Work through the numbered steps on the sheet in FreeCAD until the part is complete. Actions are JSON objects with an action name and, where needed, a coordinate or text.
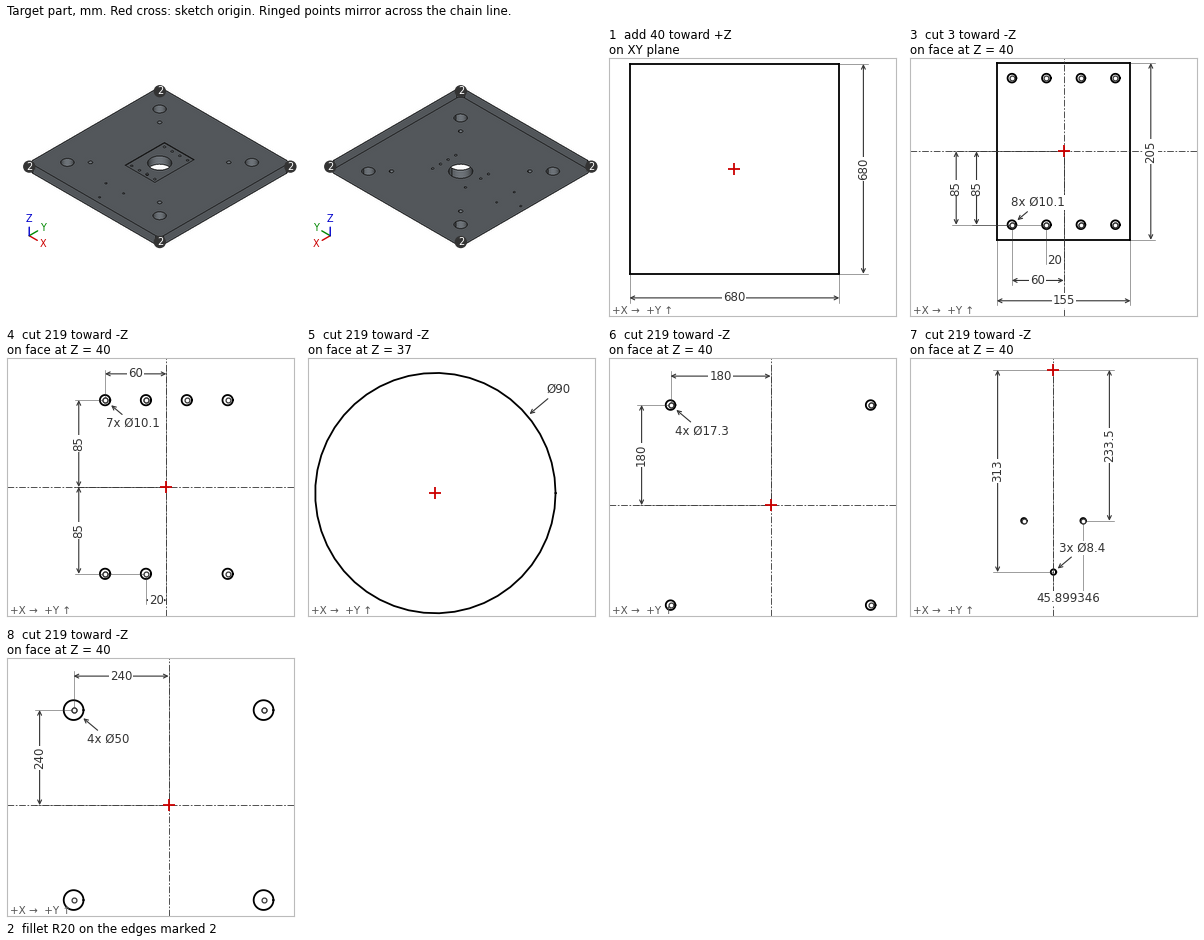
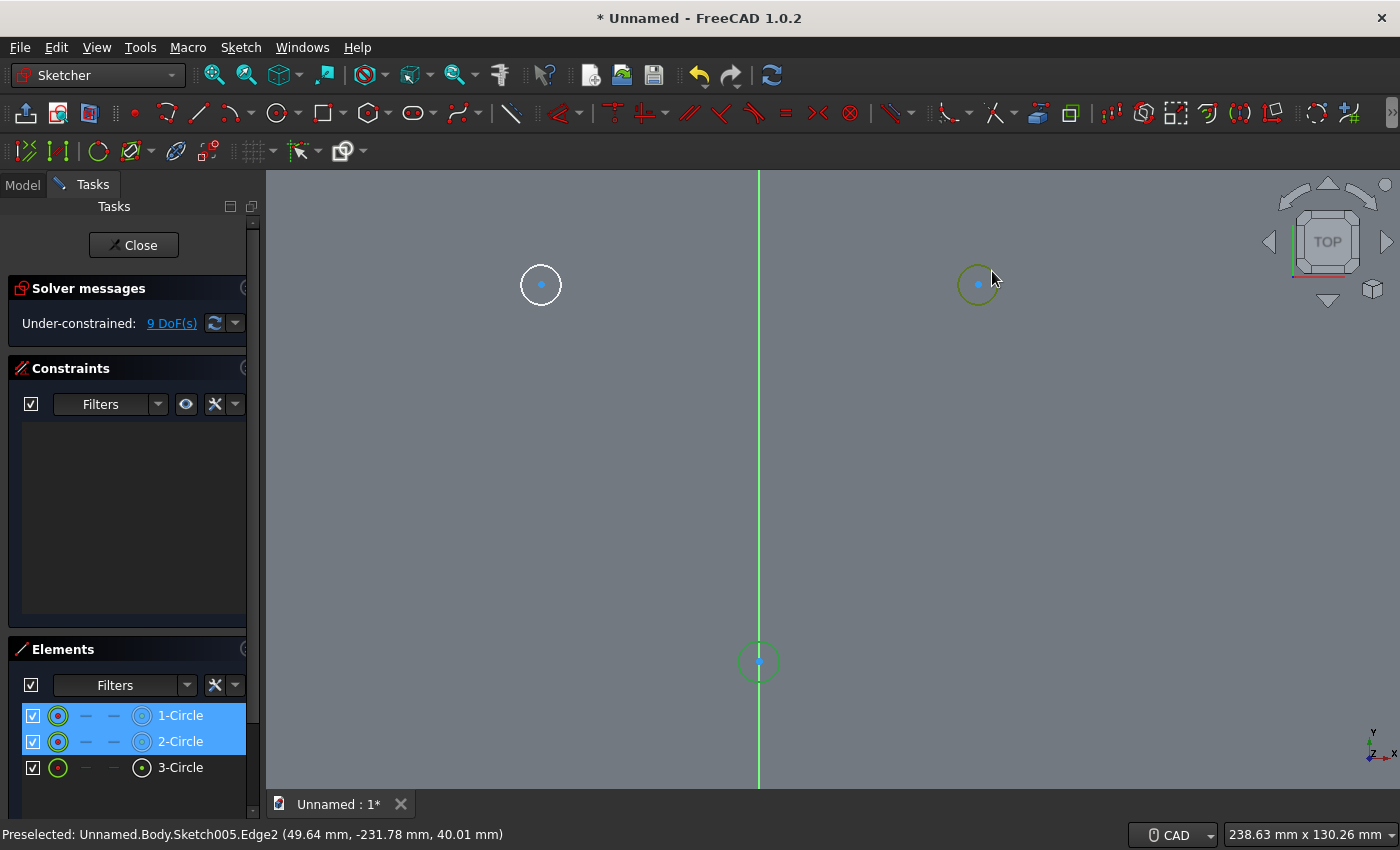
{"action": "left_click", "coordinate": [555, 271]}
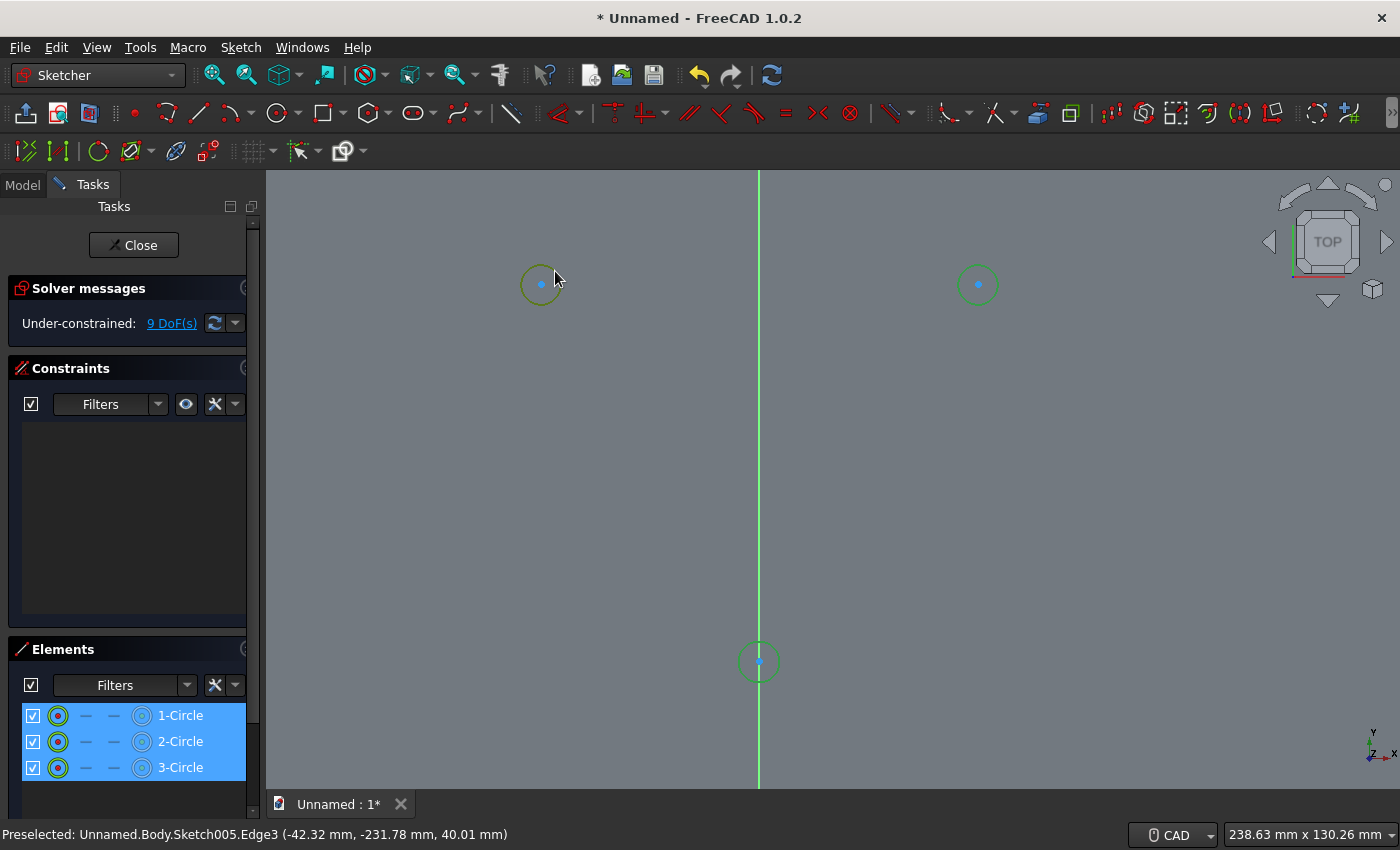
{"action": "left_click", "coordinate": [786, 114]}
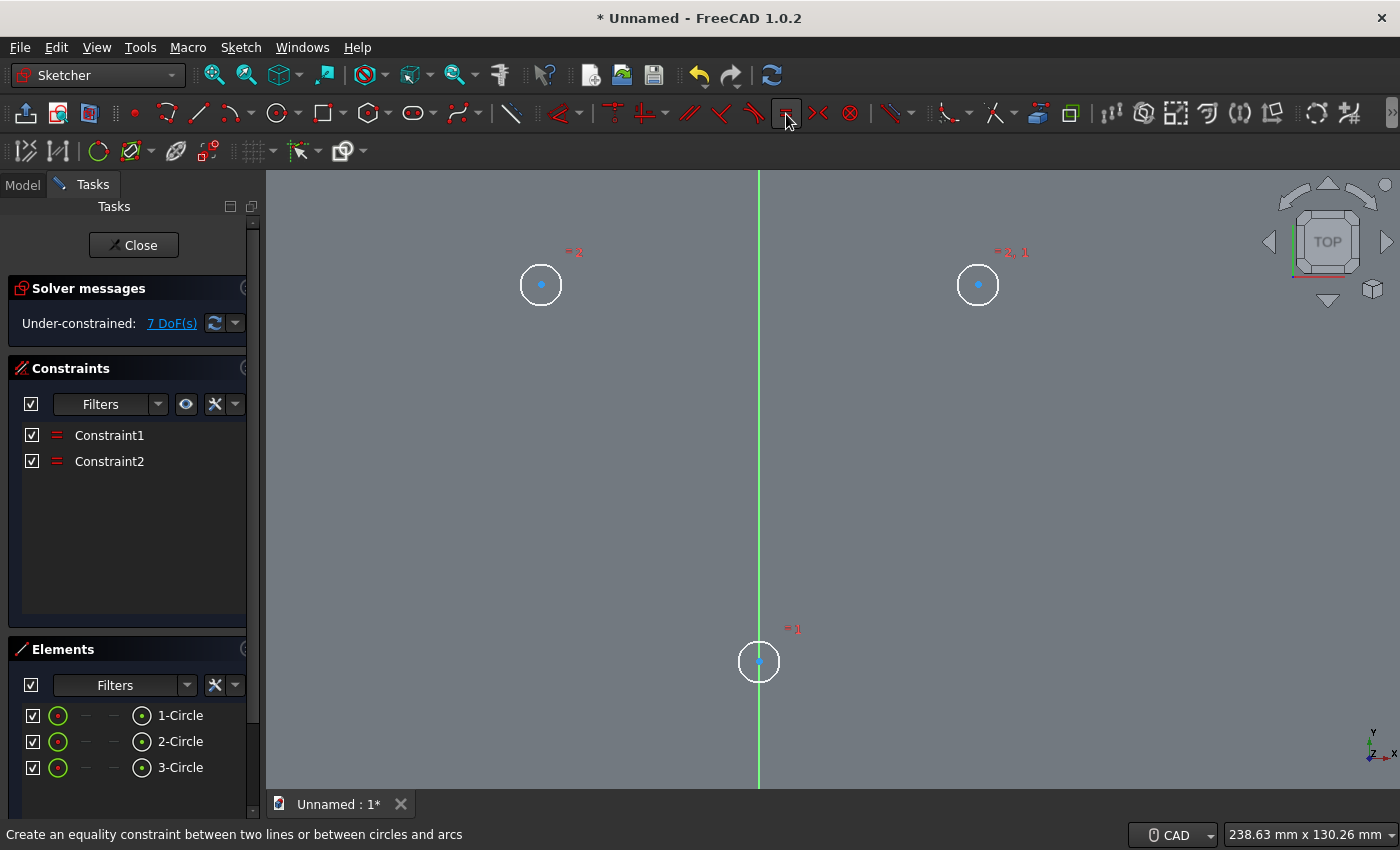
{"action": "left_click", "coordinate": [759, 662]}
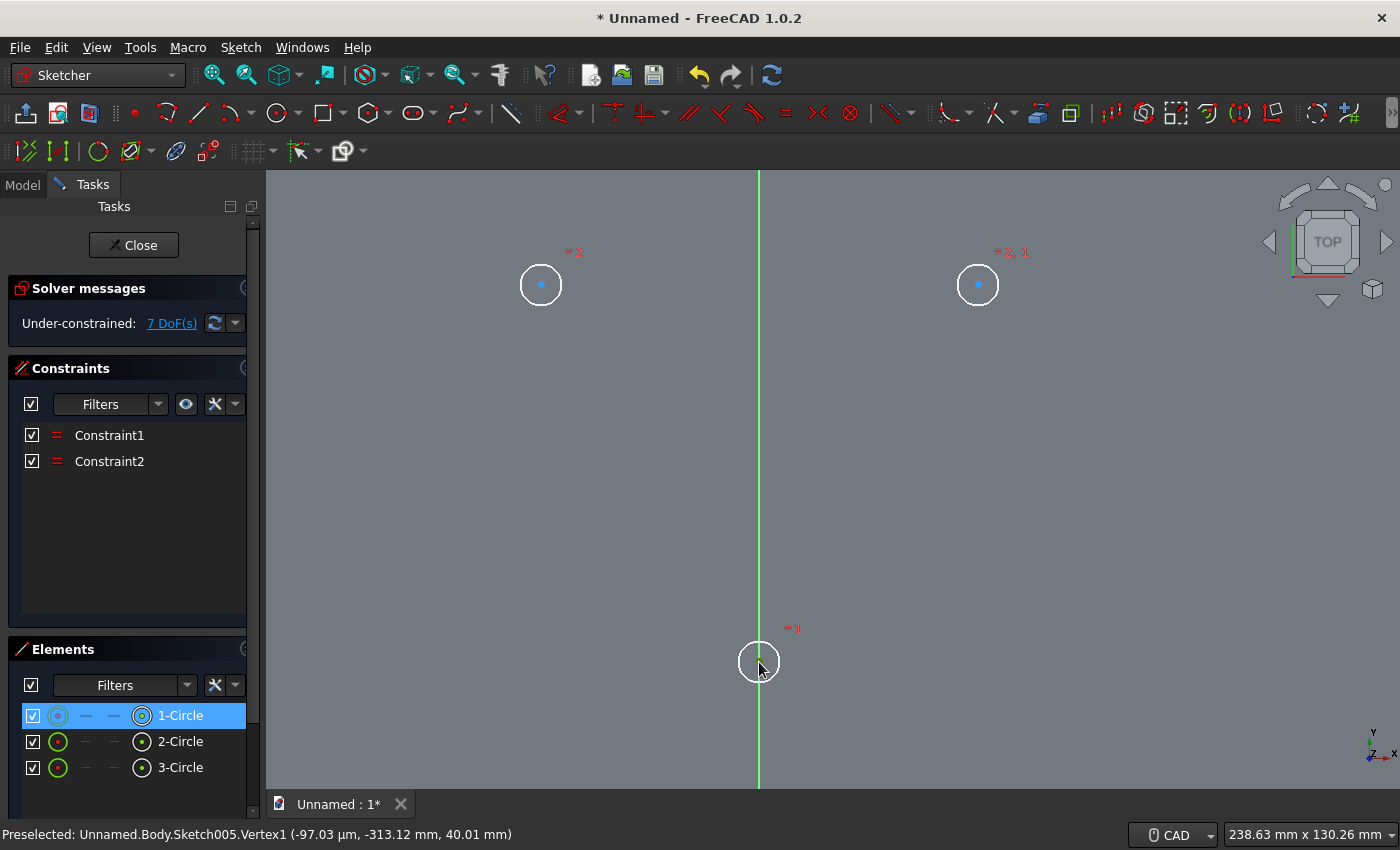
{"action": "left_click", "coordinate": [759, 721]}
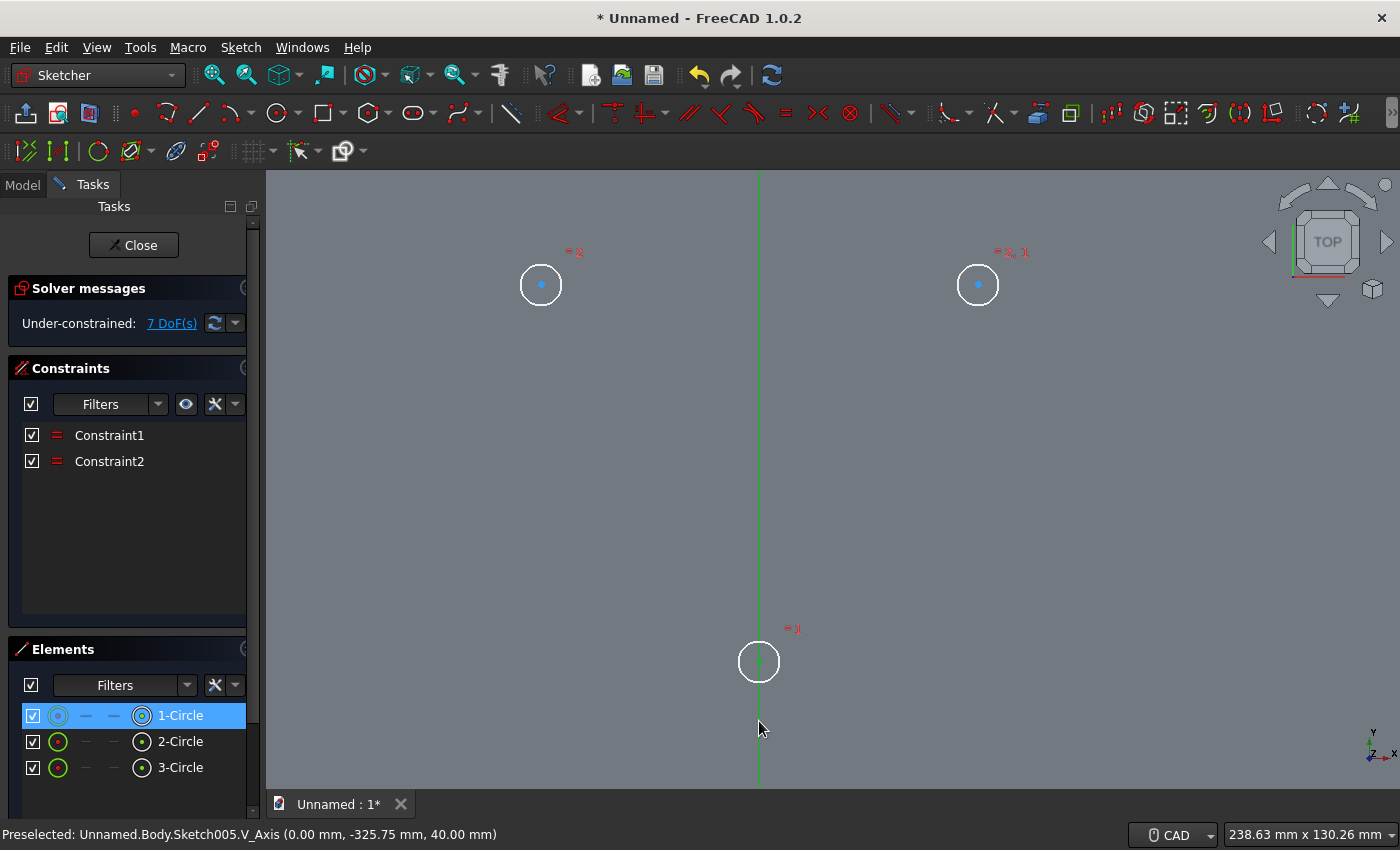
{"action": "left_click", "coordinate": [614, 114]}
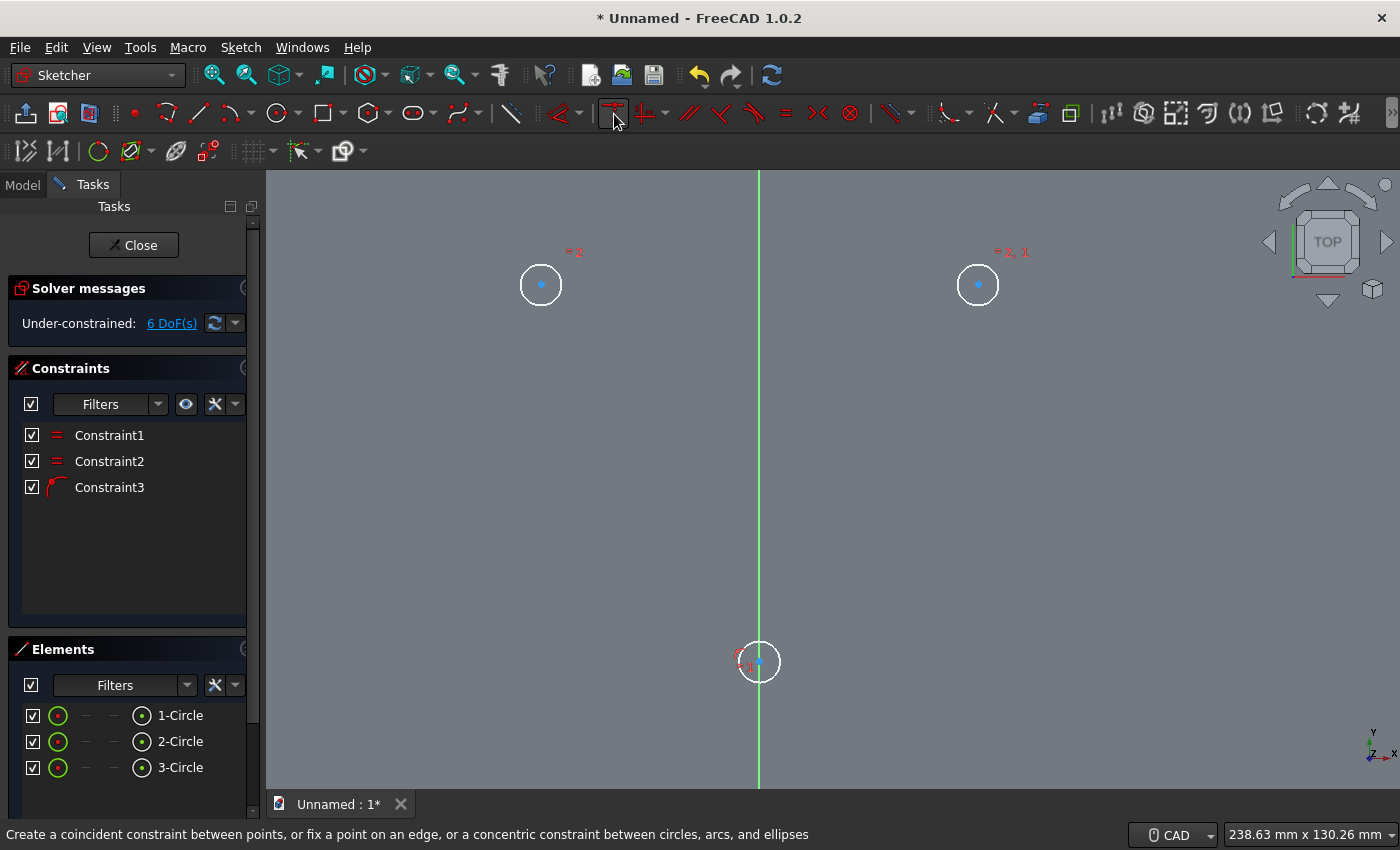
{"action": "left_click", "coordinate": [978, 285]}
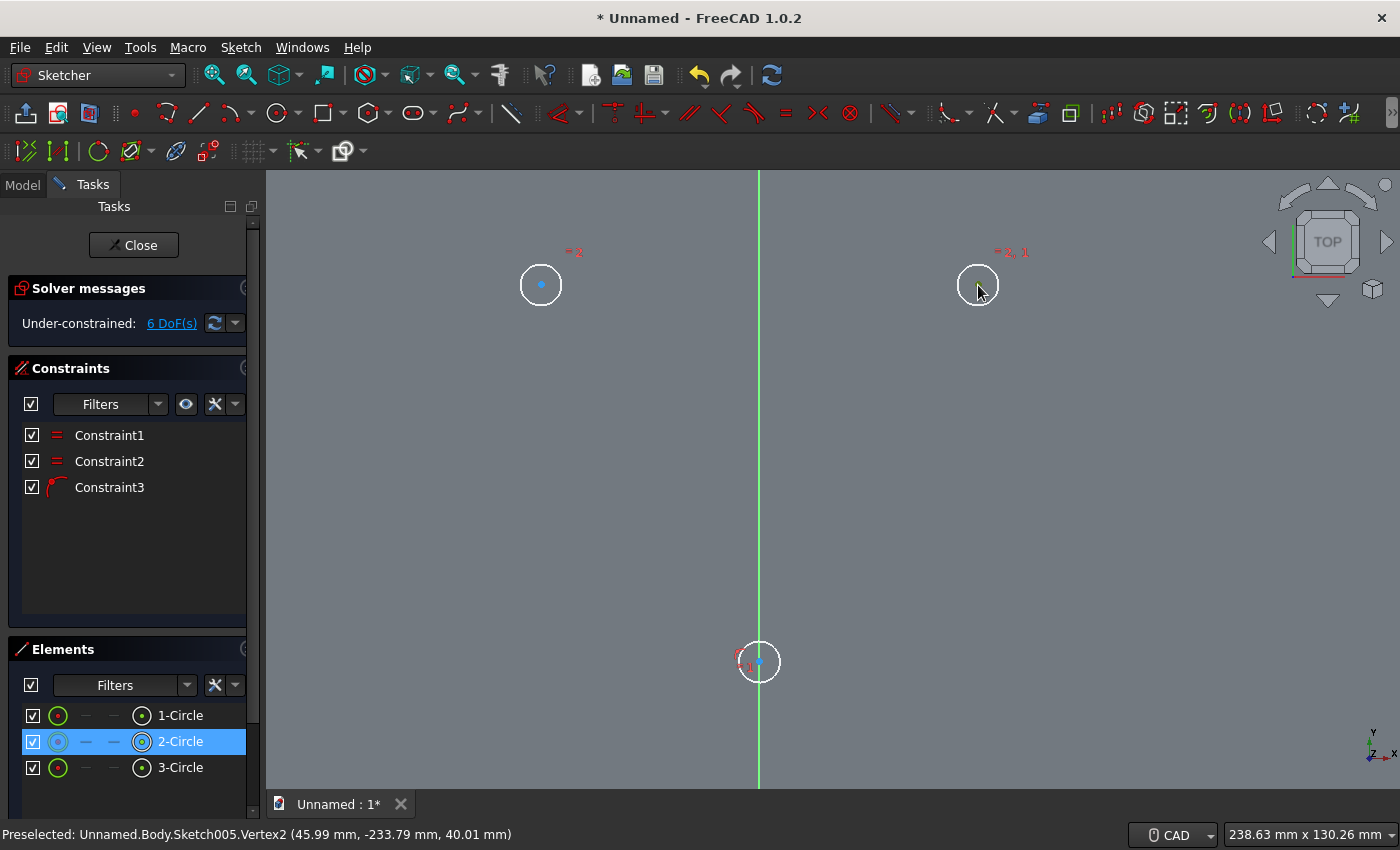
{"action": "left_click", "coordinate": [541, 285]}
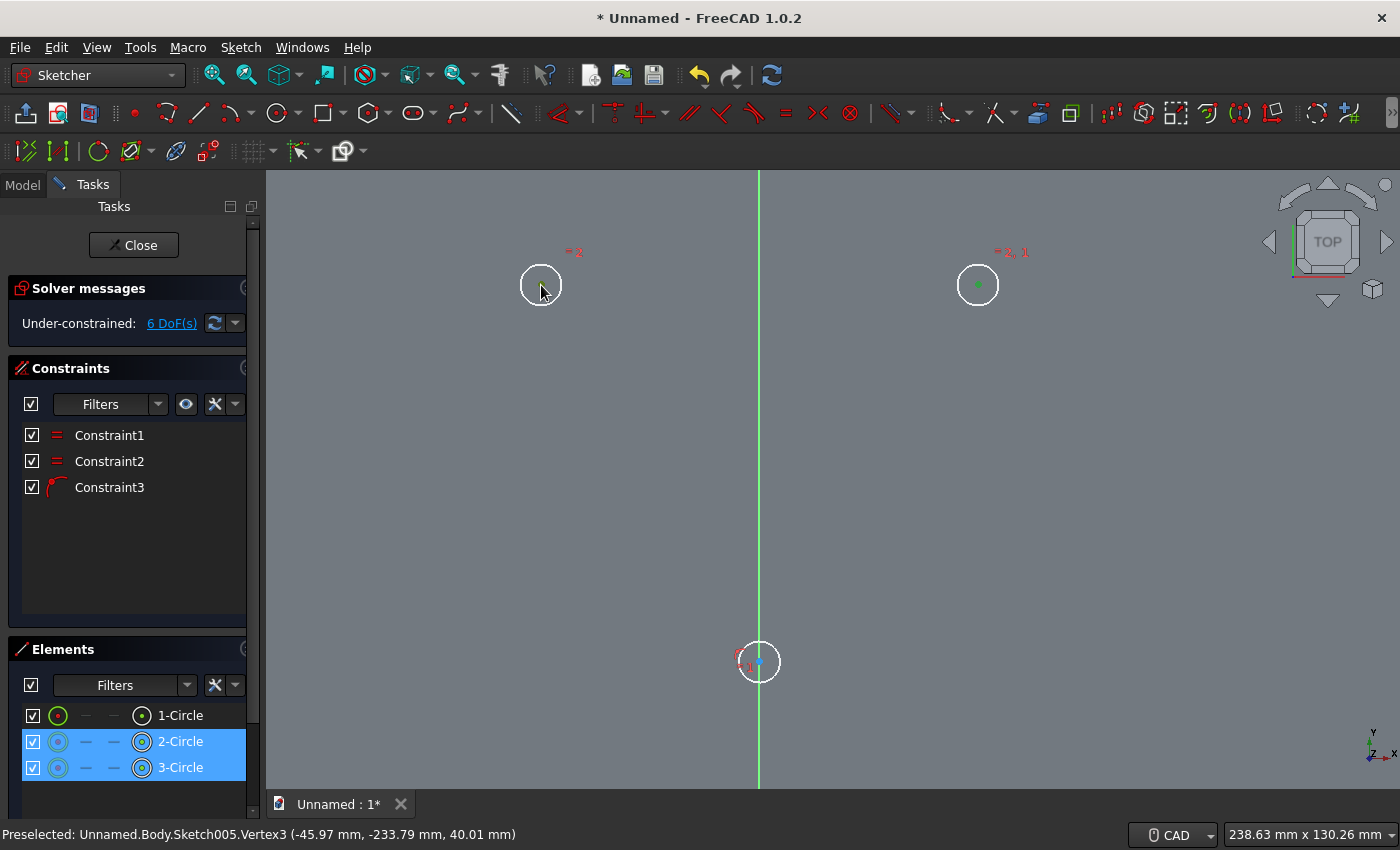
{"action": "left_click", "coordinate": [759, 721]}